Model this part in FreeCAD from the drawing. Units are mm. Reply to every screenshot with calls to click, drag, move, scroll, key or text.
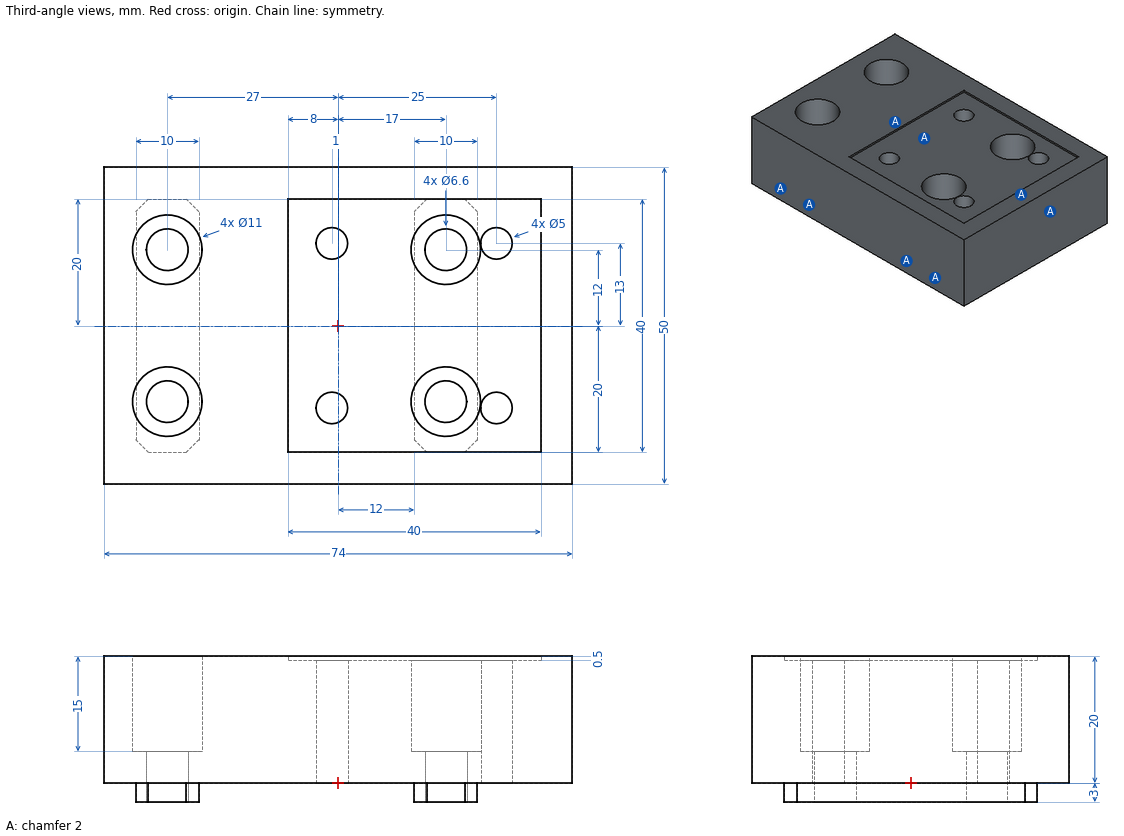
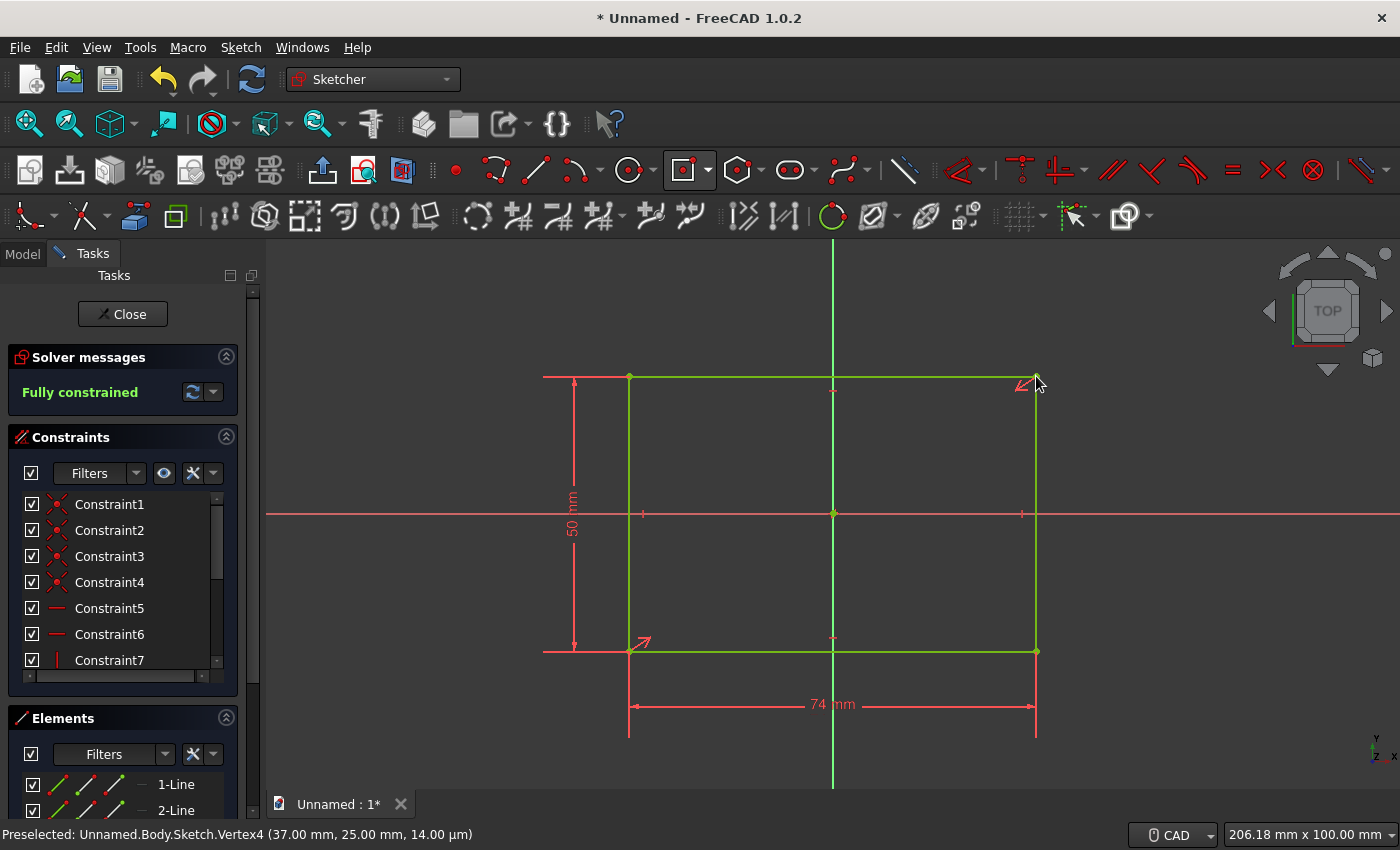
click(123, 314)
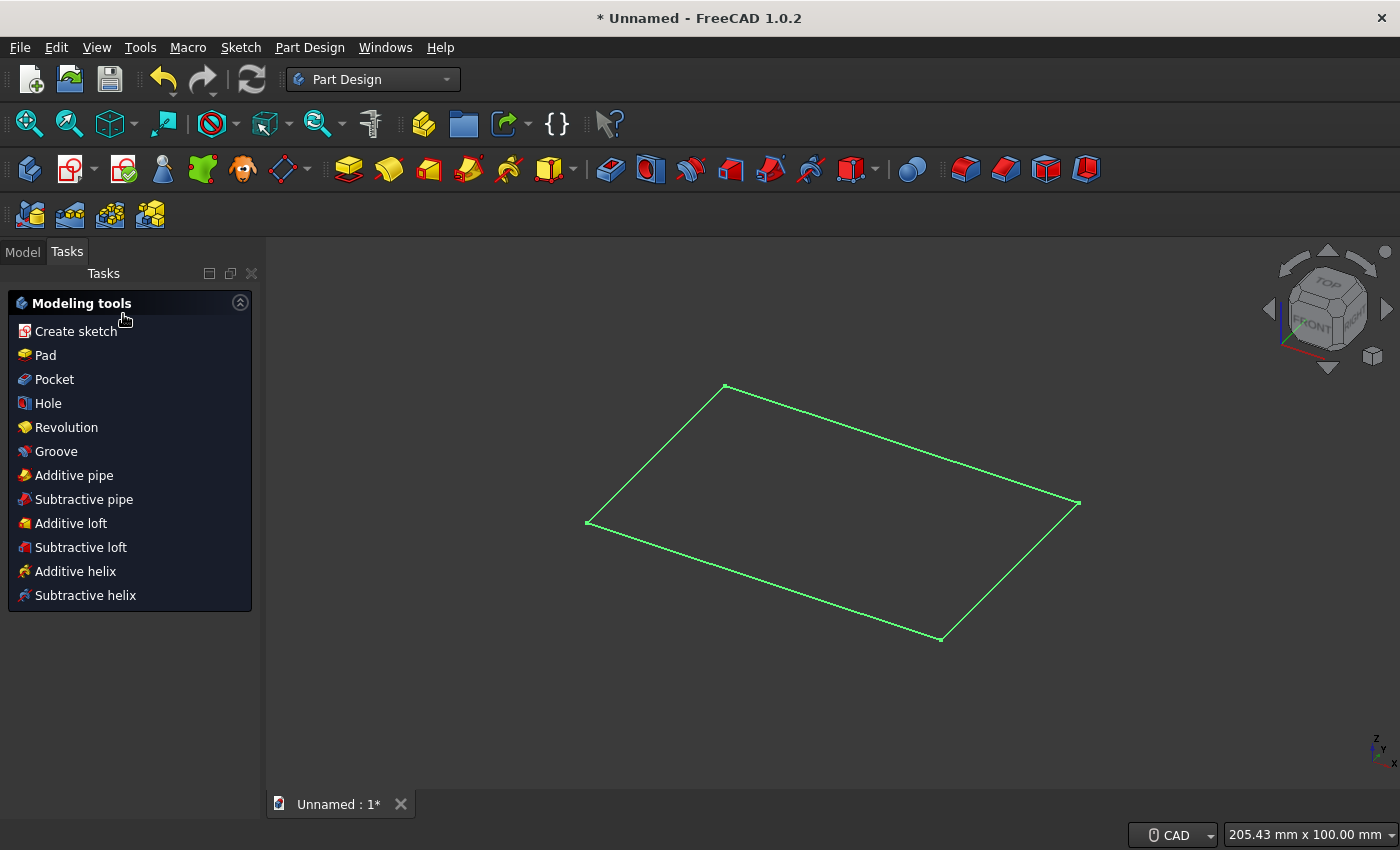
click(350, 170)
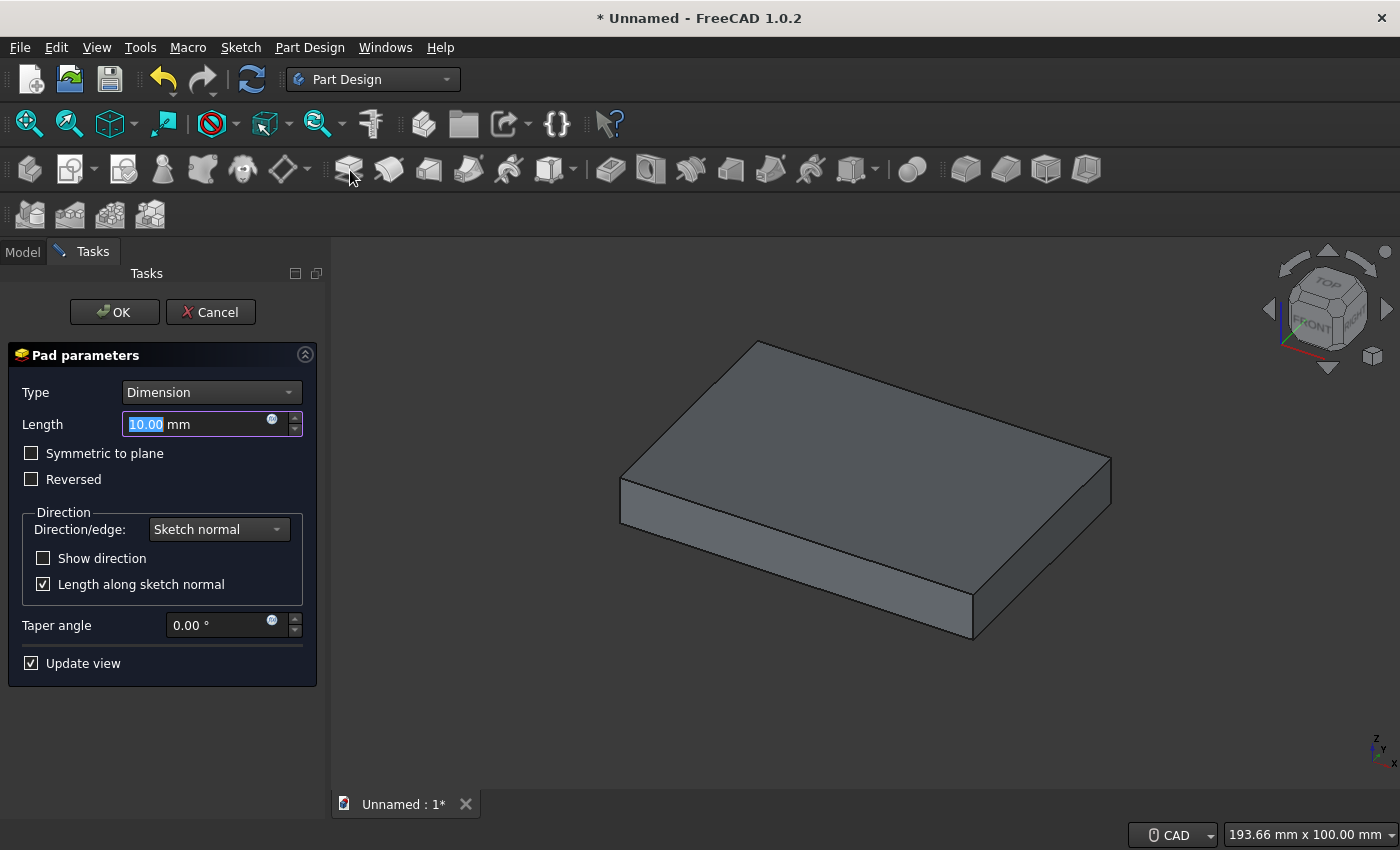
text(20)
key(Tab)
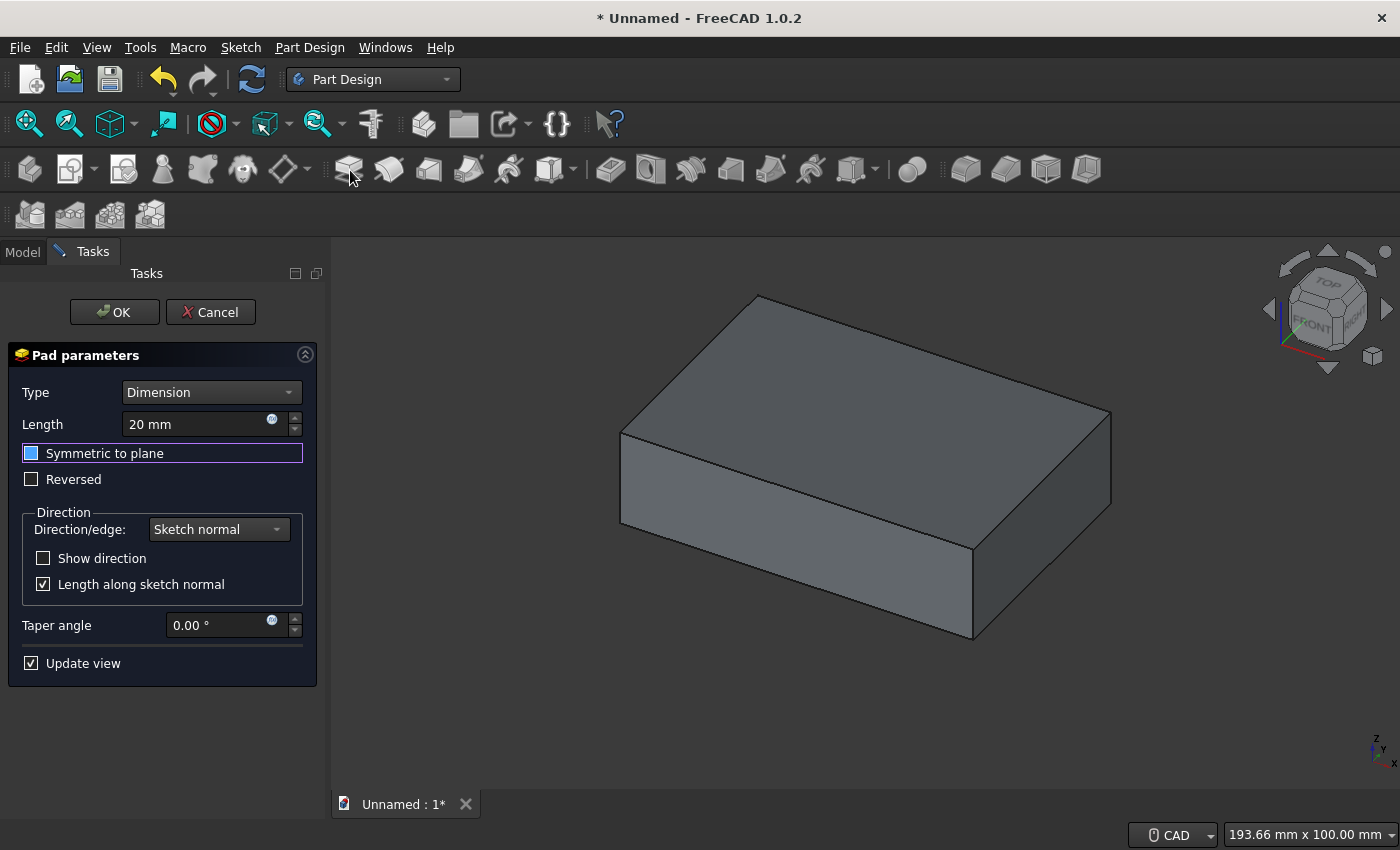
click(115, 312)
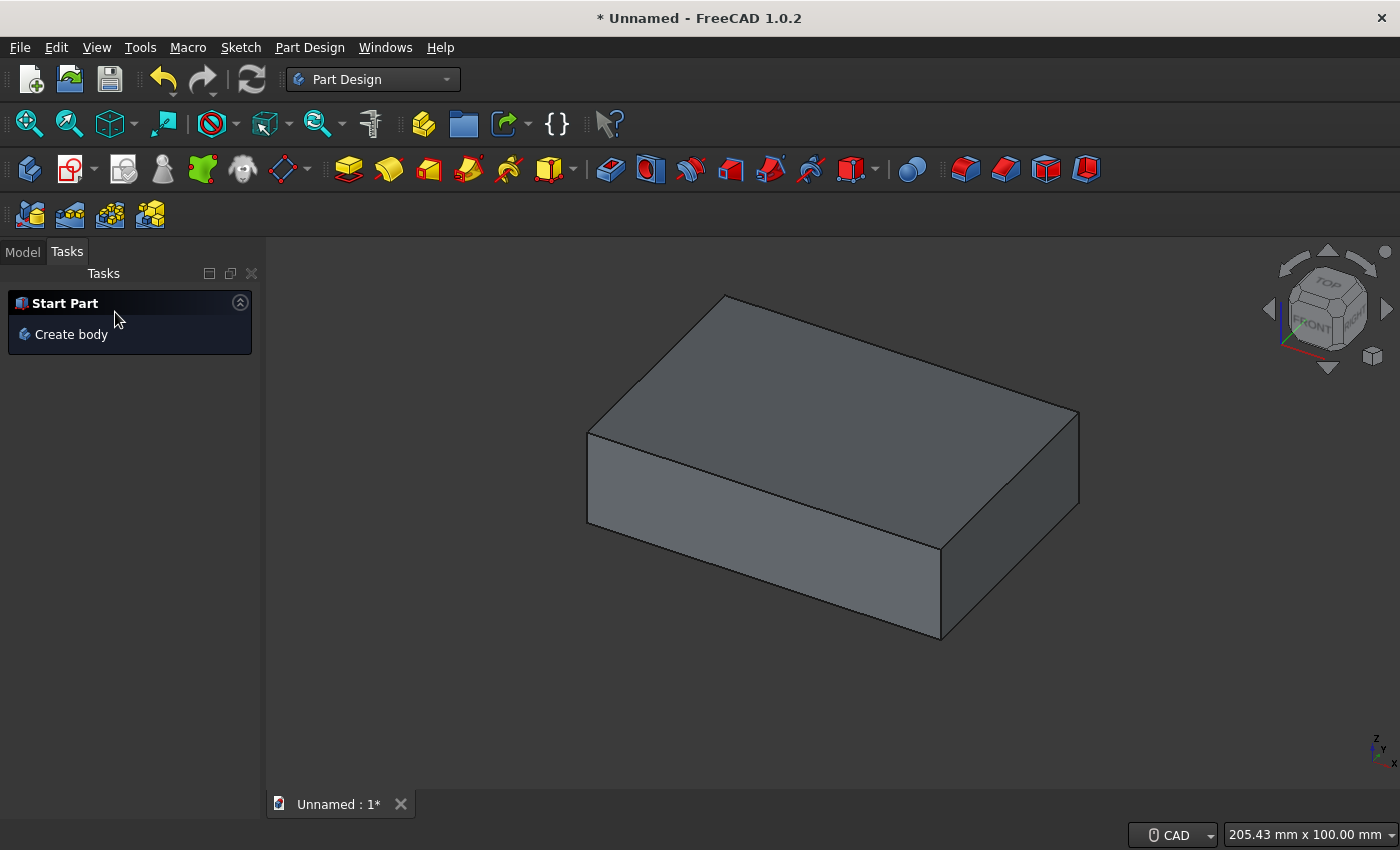
click(884, 438)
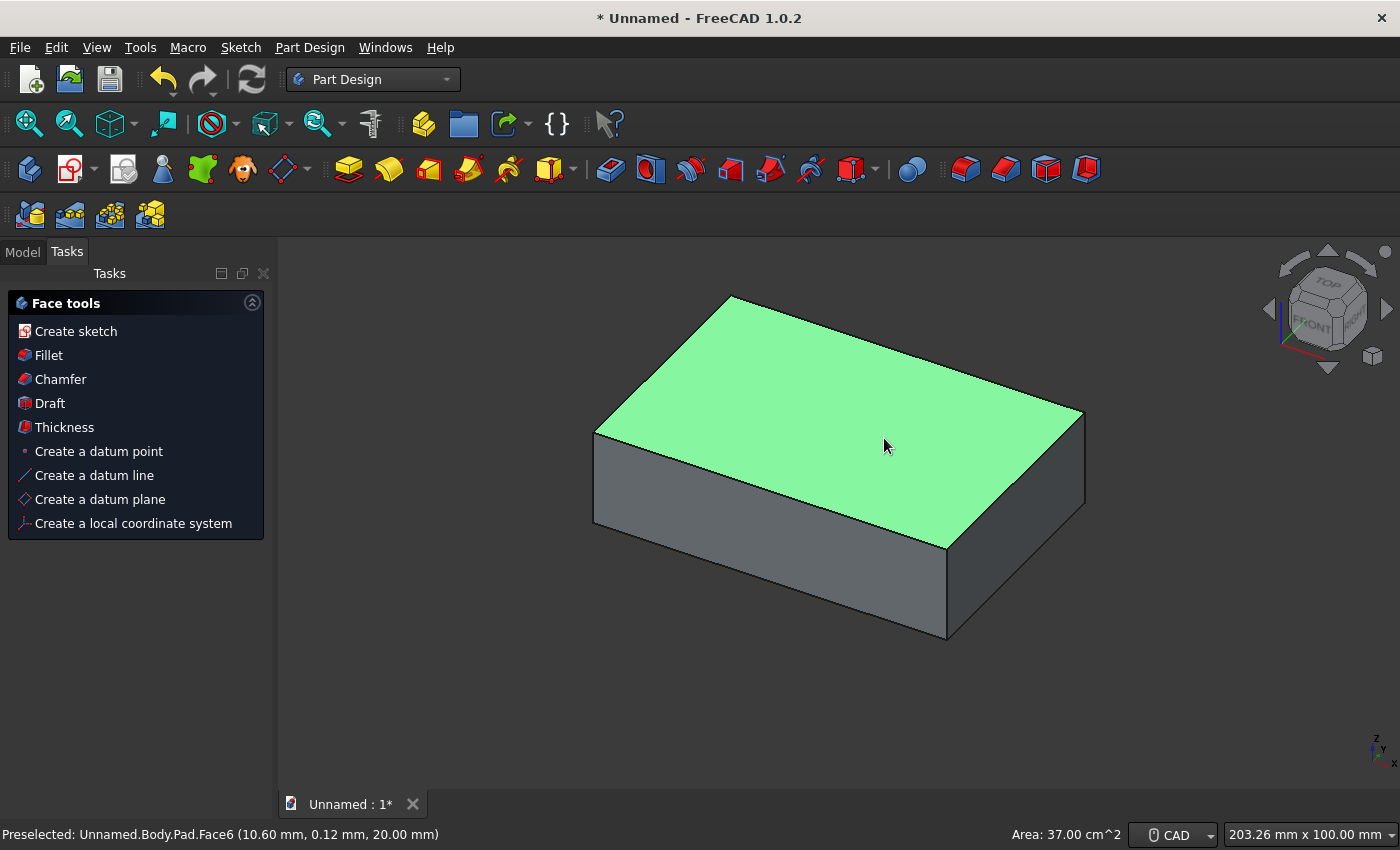
click(70, 170)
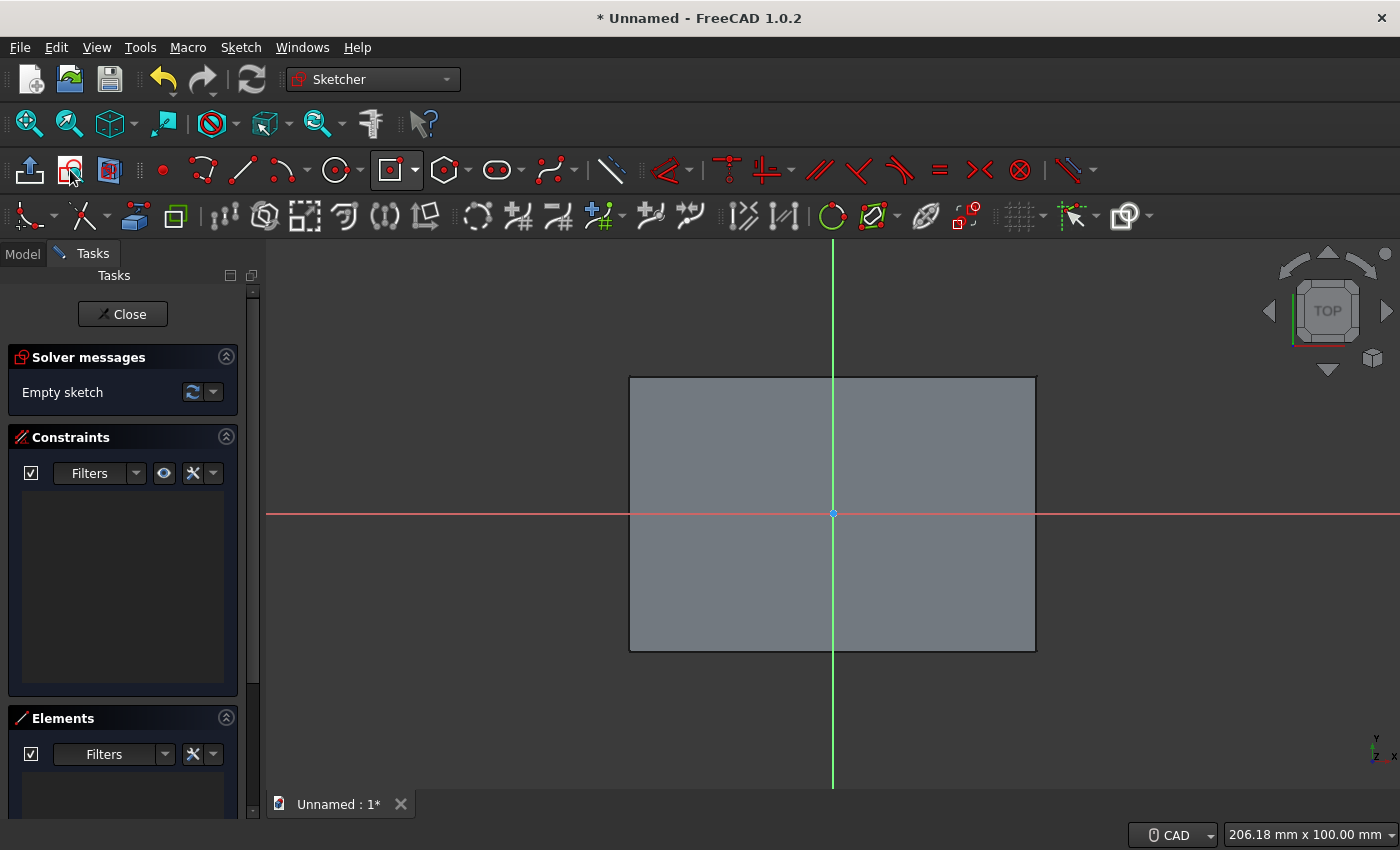
scroll(1172, 514, up, 2)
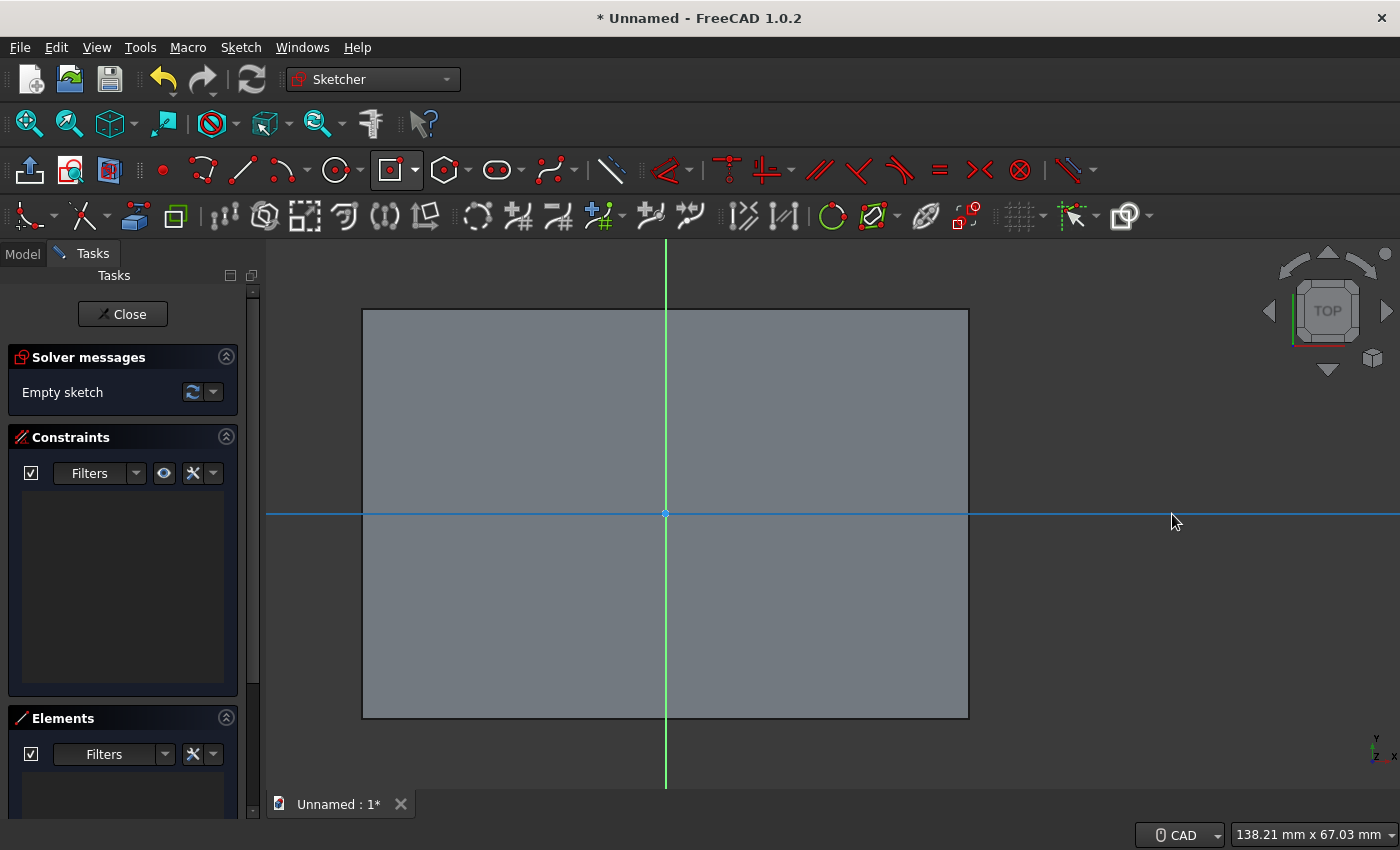
click(418, 170)